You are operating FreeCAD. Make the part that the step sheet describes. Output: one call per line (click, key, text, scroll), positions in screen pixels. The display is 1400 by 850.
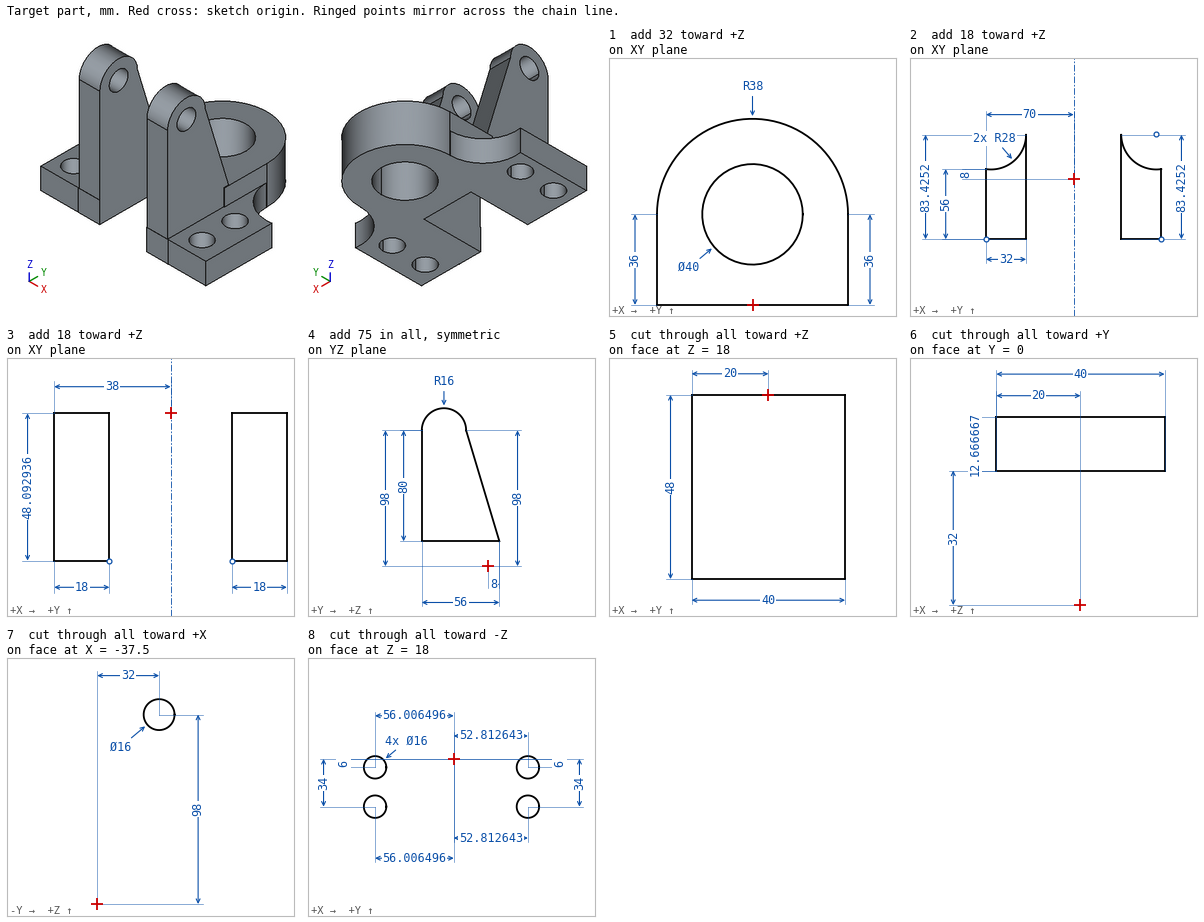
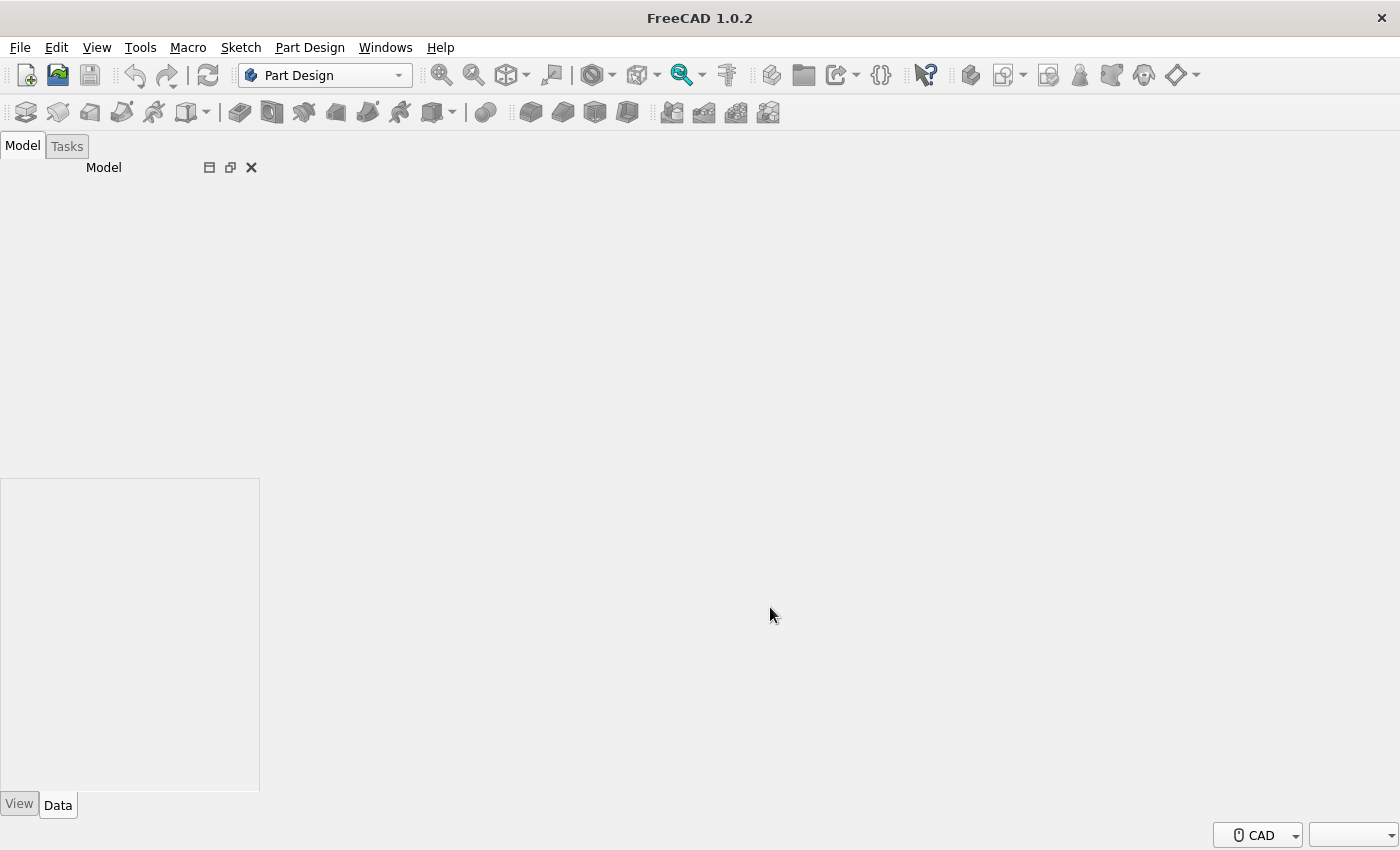
click(26, 76)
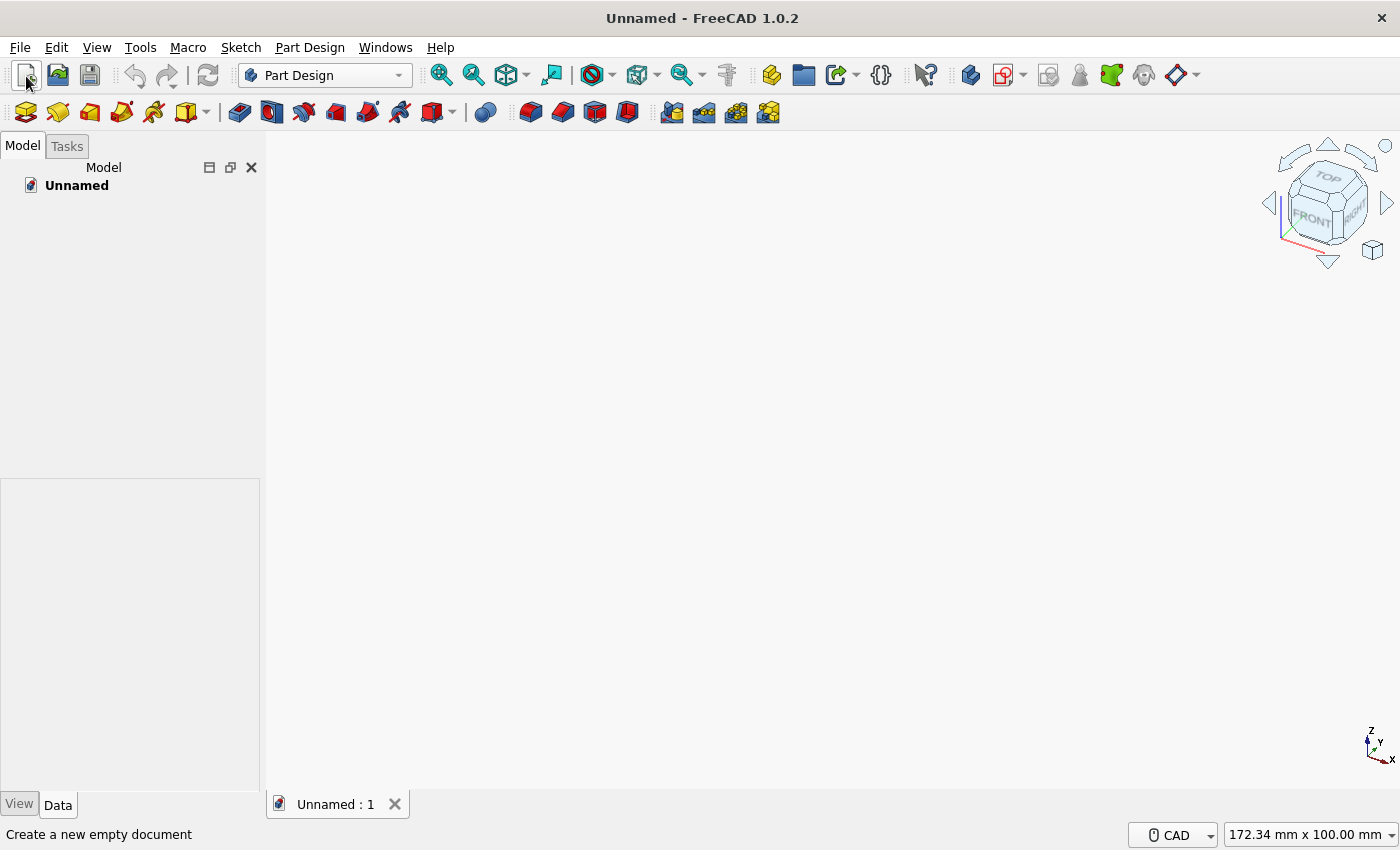
click(1004, 76)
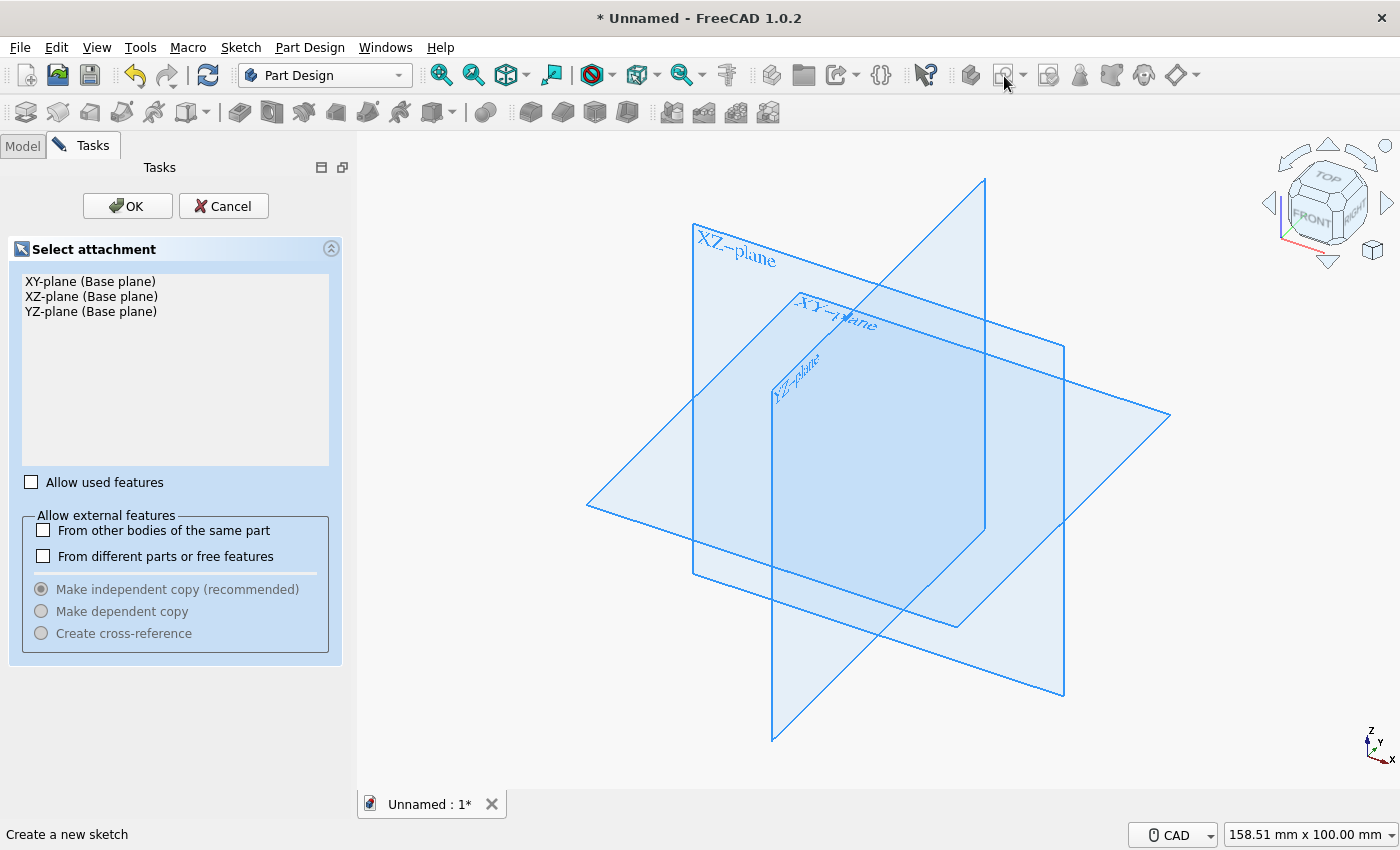
click(82, 282)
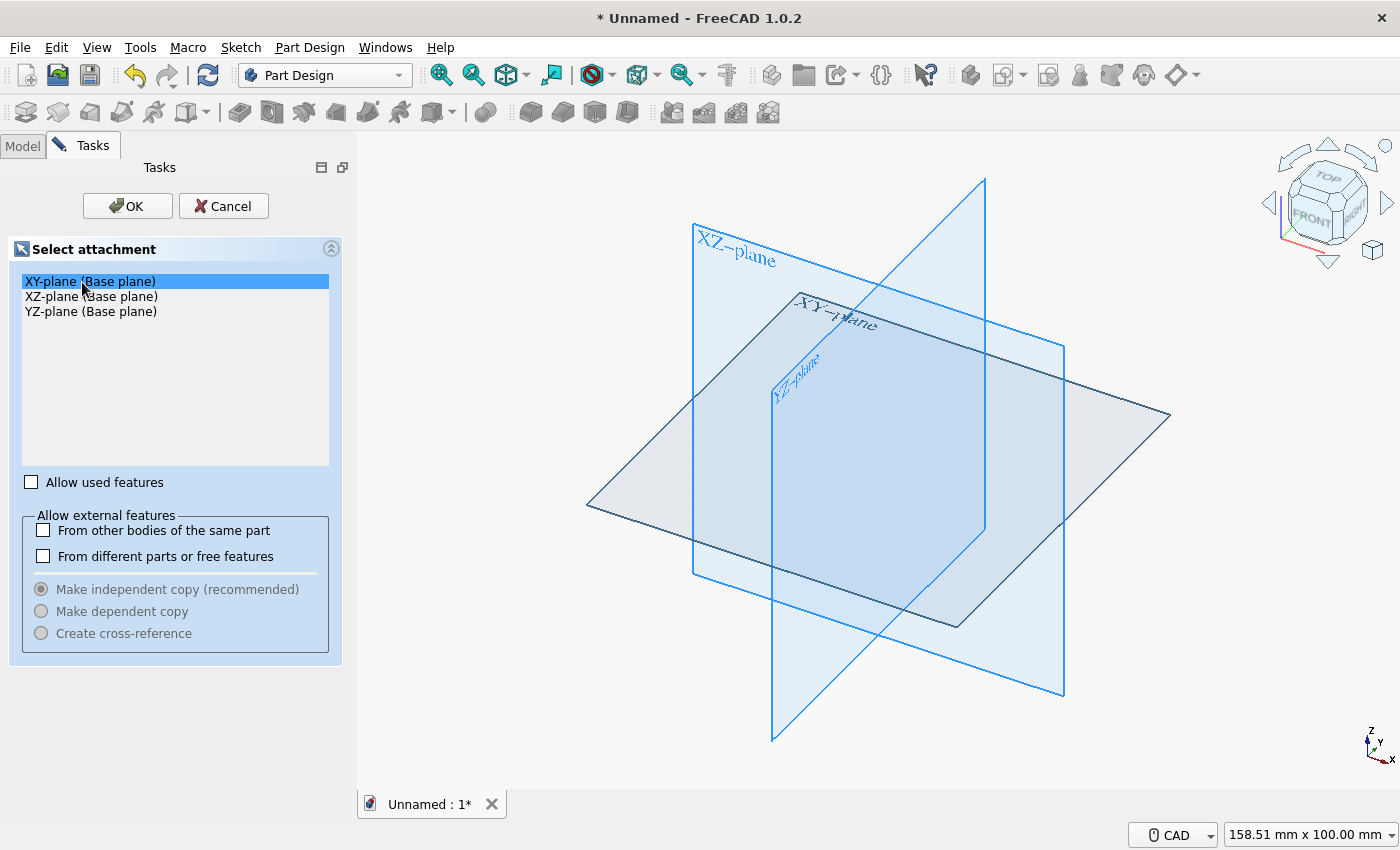
click(128, 206)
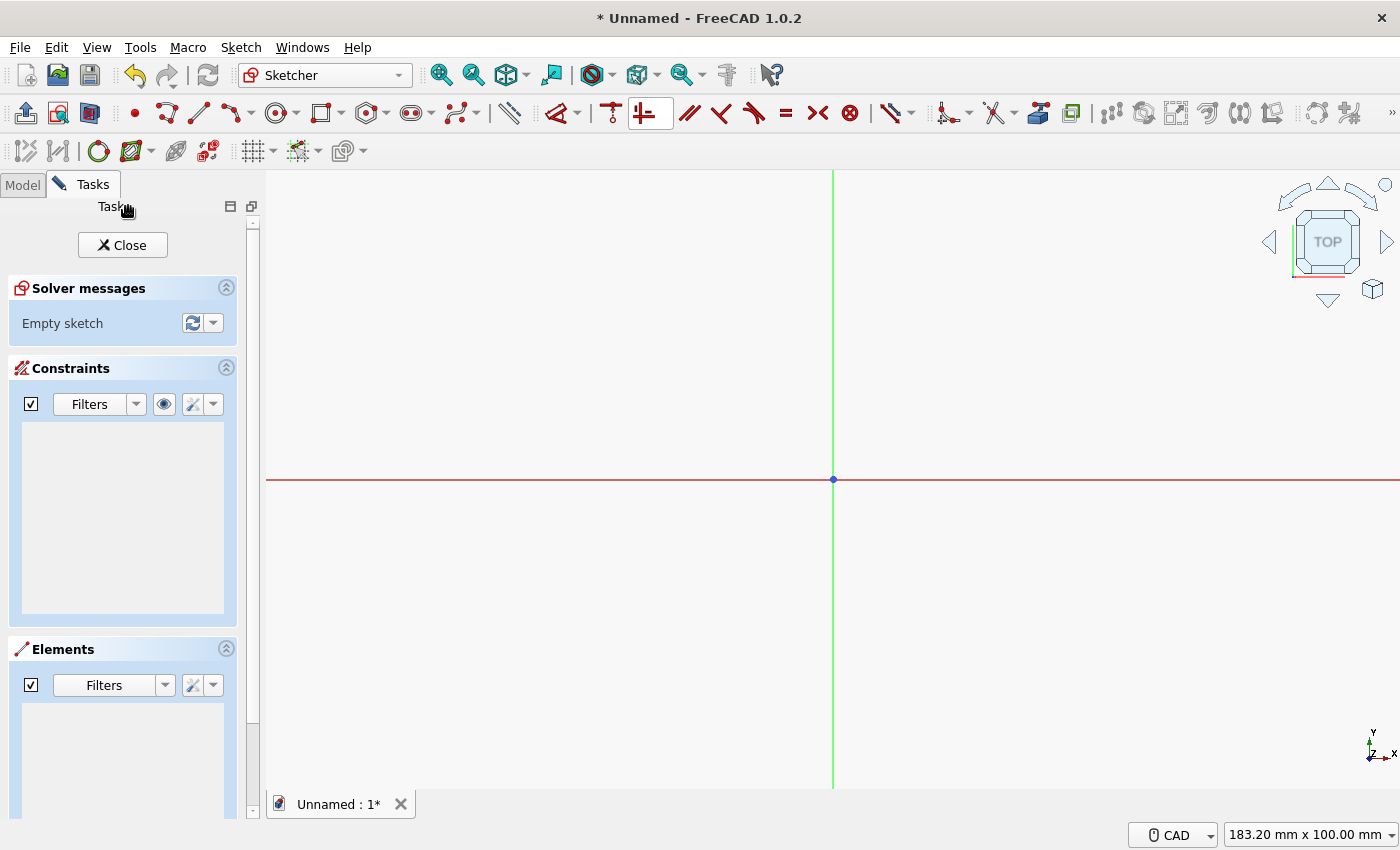
scroll(625, 761, down, 2)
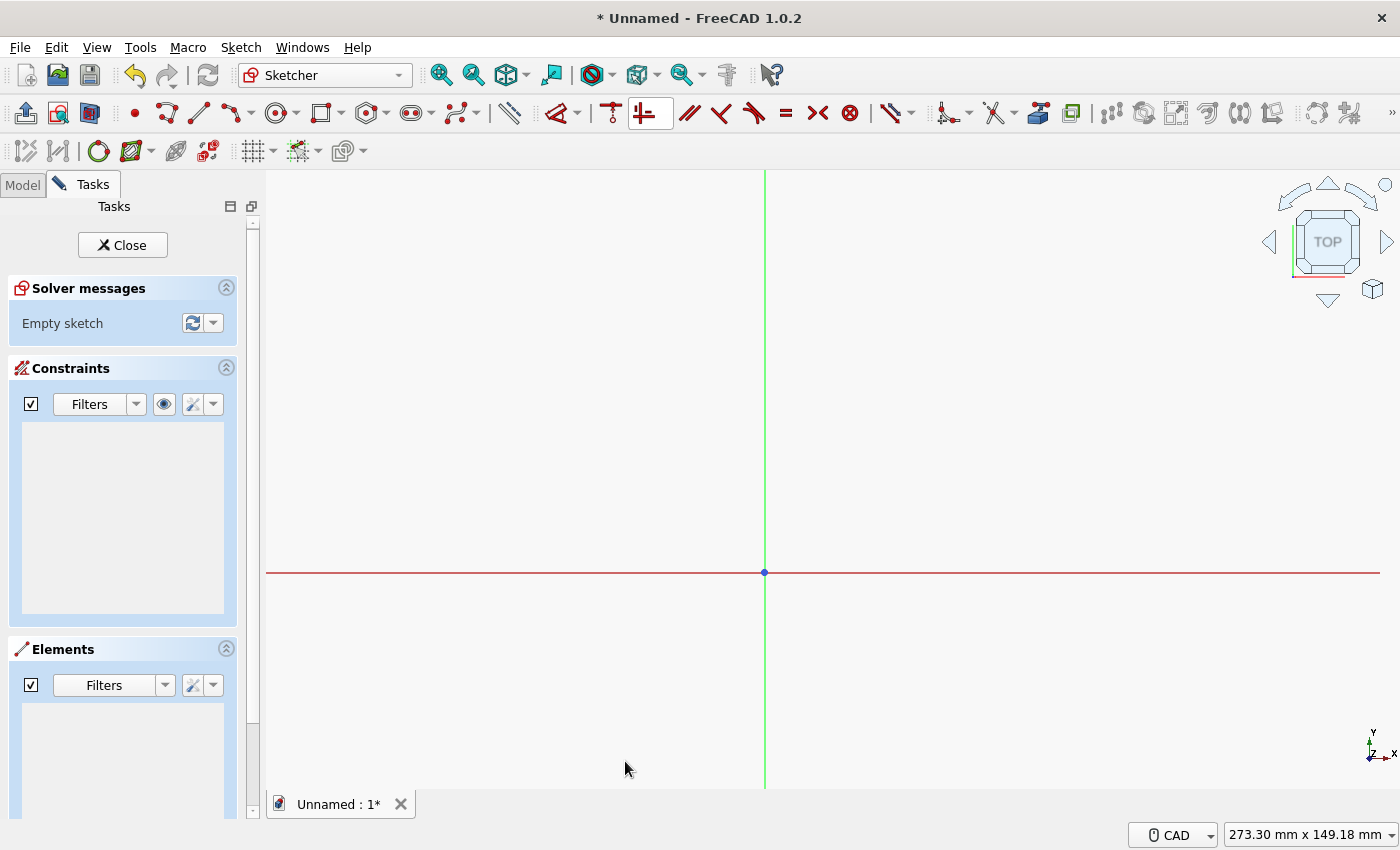
click(168, 114)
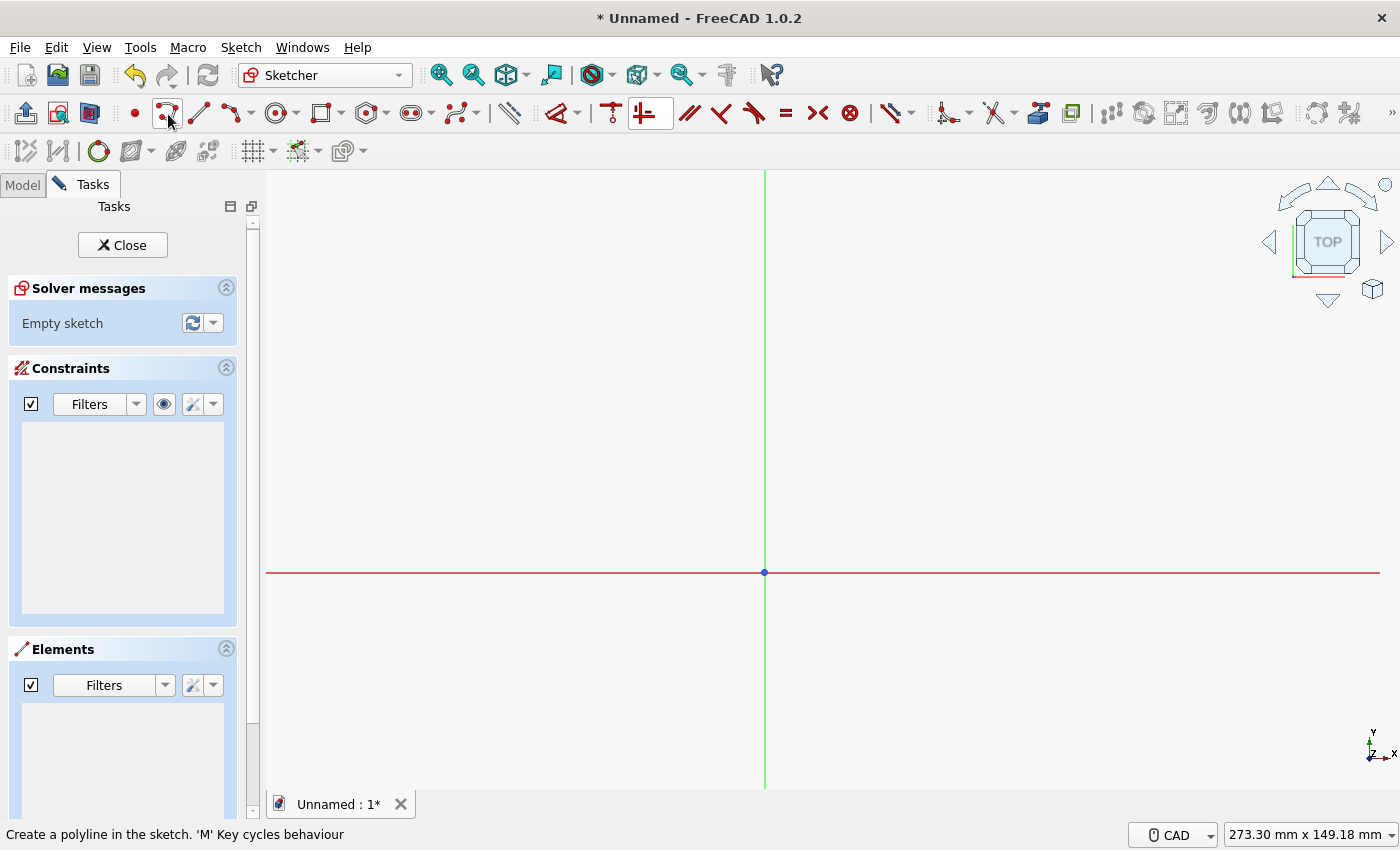
click(607, 423)
click(607, 573)
click(922, 564)
click(922, 423)
right_click(922, 423)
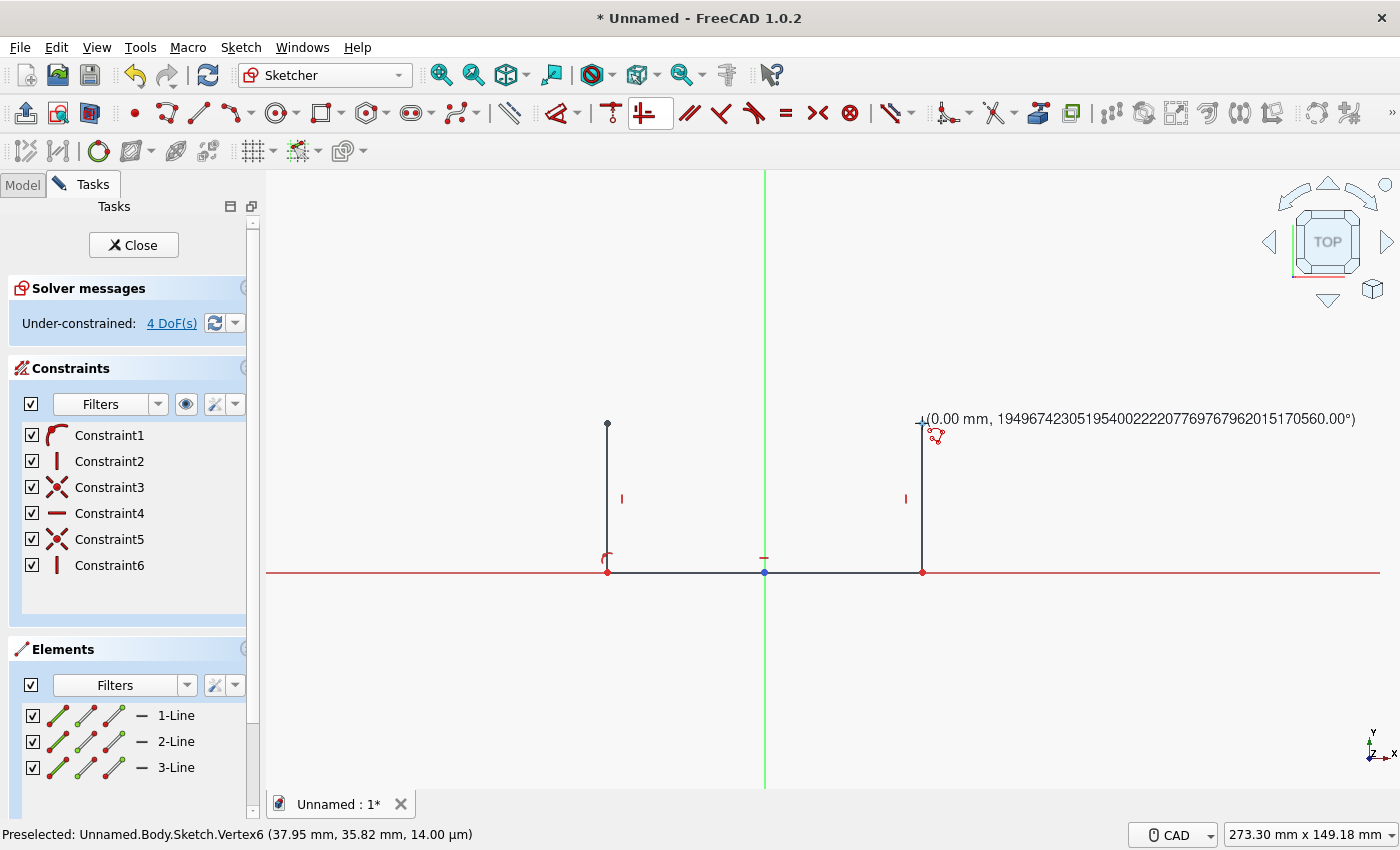
click(232, 114)